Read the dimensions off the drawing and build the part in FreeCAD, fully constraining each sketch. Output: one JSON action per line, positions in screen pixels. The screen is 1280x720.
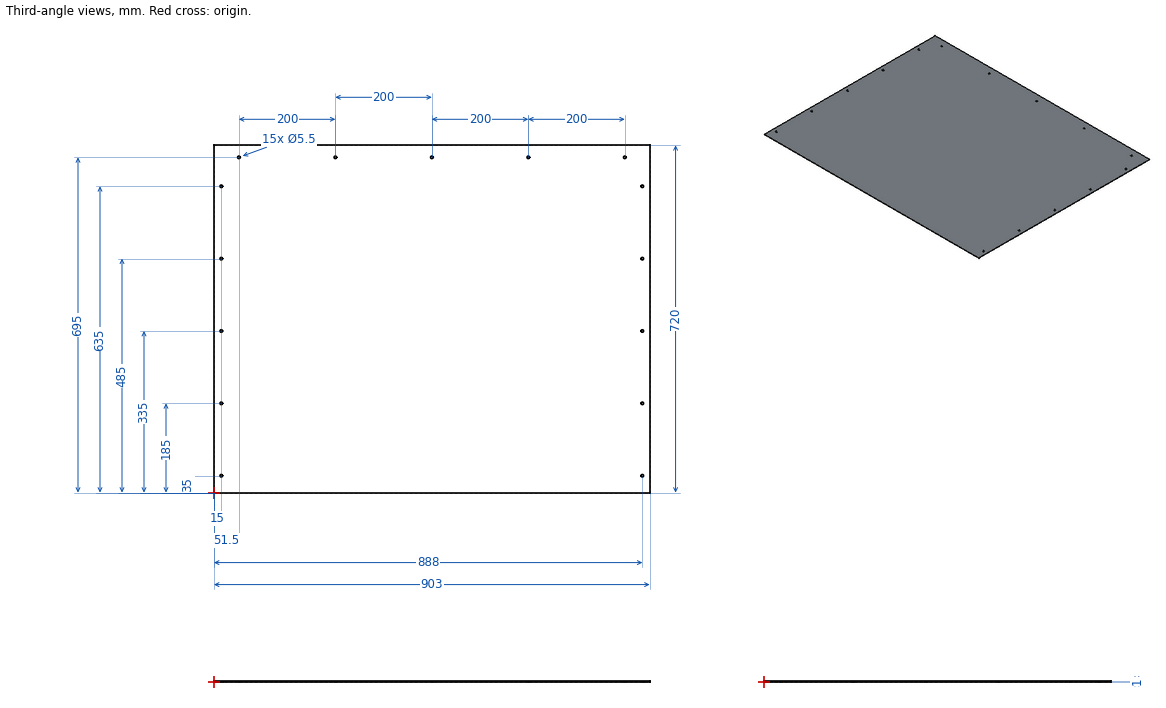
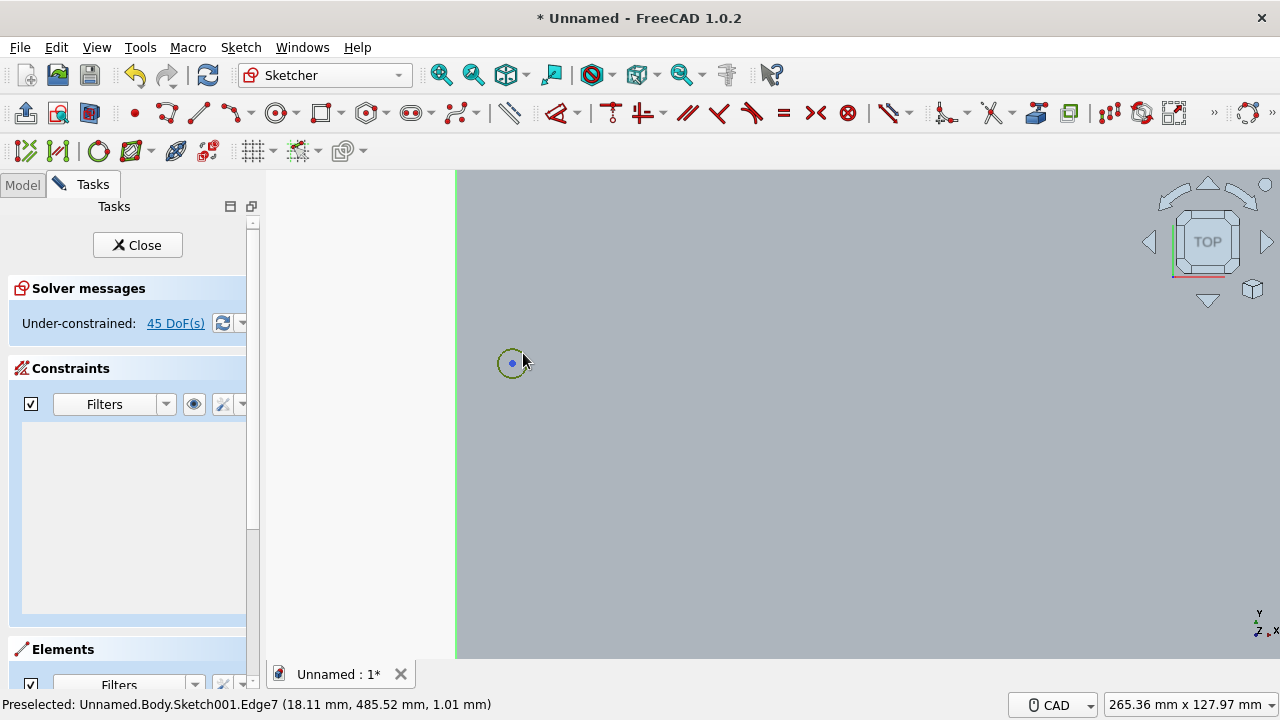
{"action": "scroll", "coordinate": [523, 357], "scroll_direction": "down", "scroll_amount": 11}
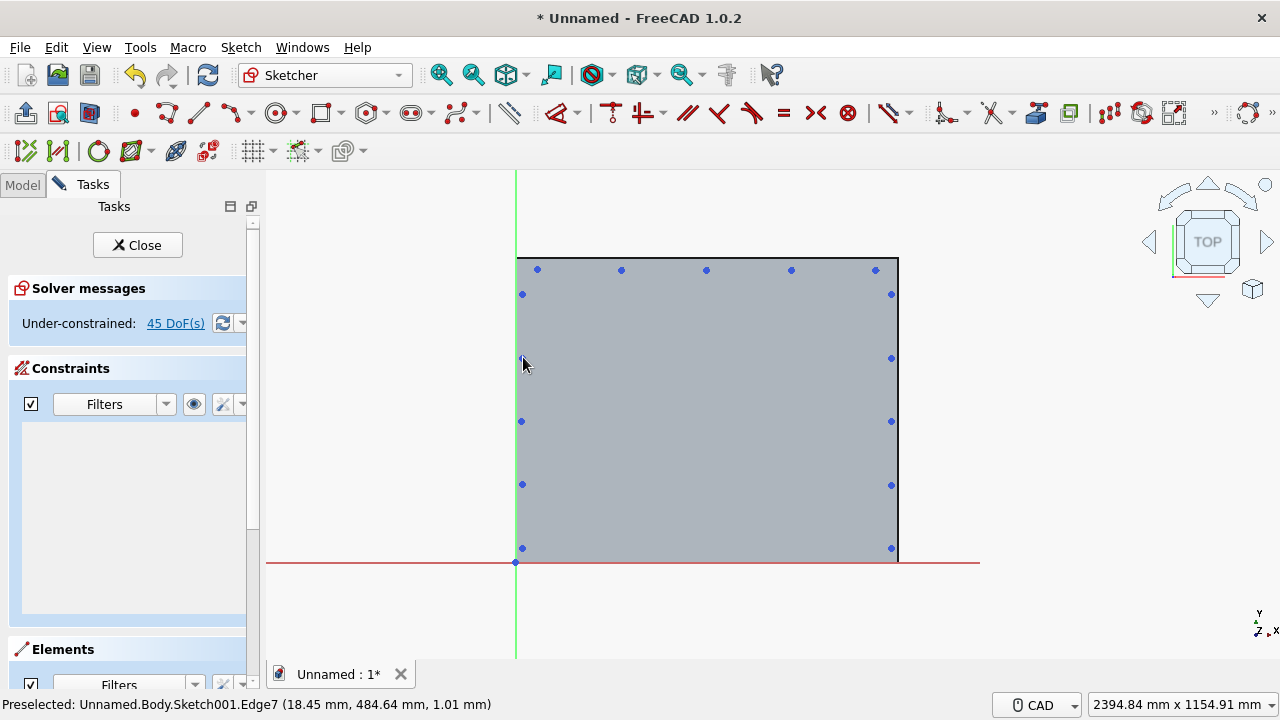
{"action": "scroll", "coordinate": [523, 420], "scroll_direction": "up", "scroll_amount": 12}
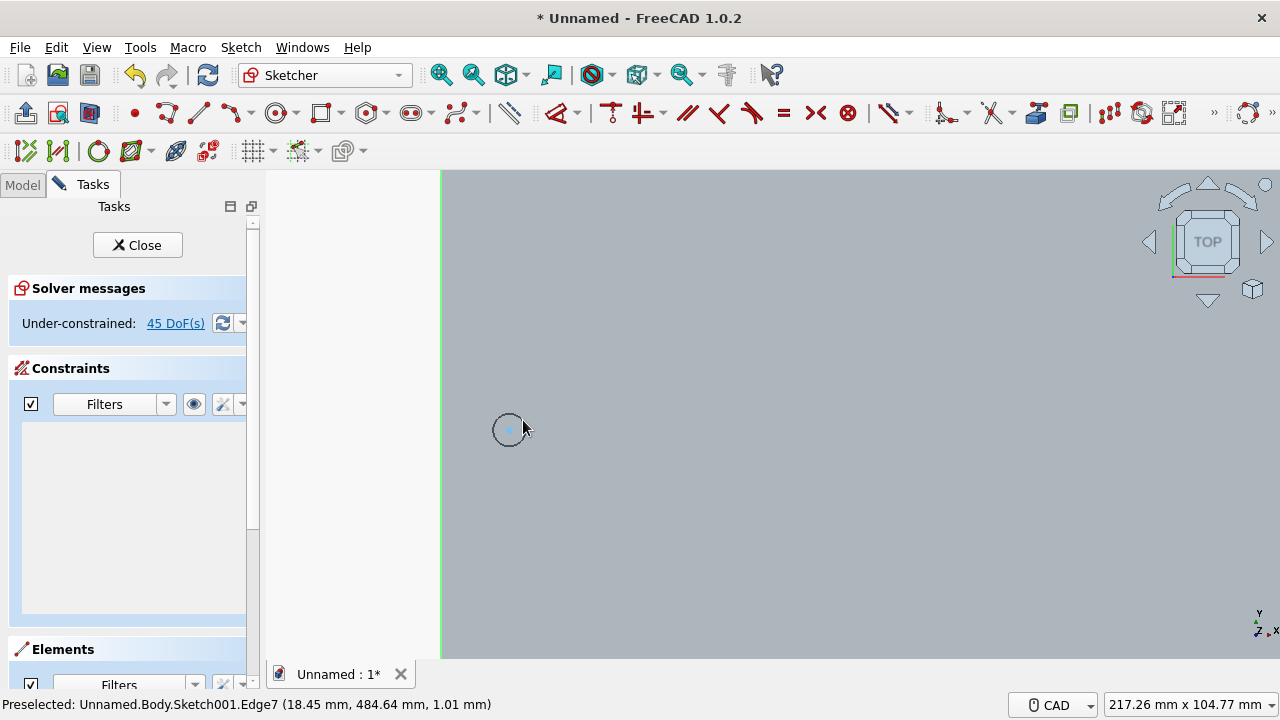
{"action": "left_click", "coordinate": [521, 419]}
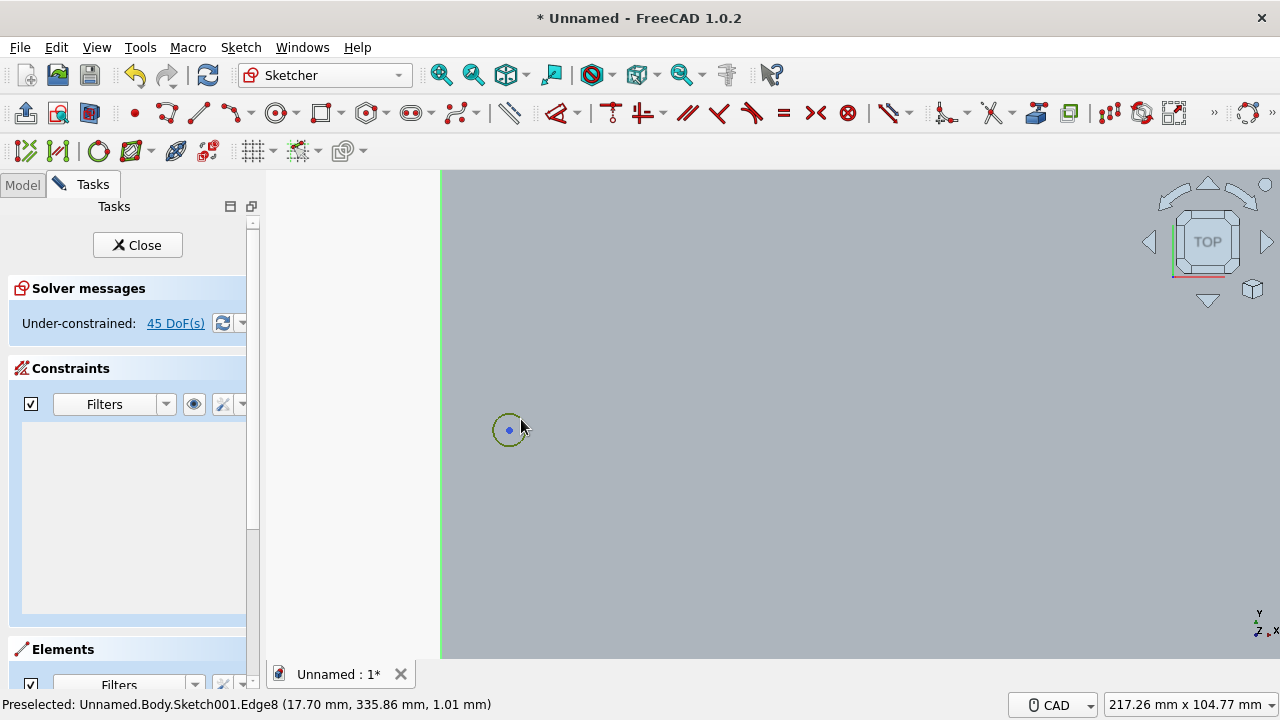
{"action": "scroll", "coordinate": [523, 420], "scroll_direction": "down", "scroll_amount": 12}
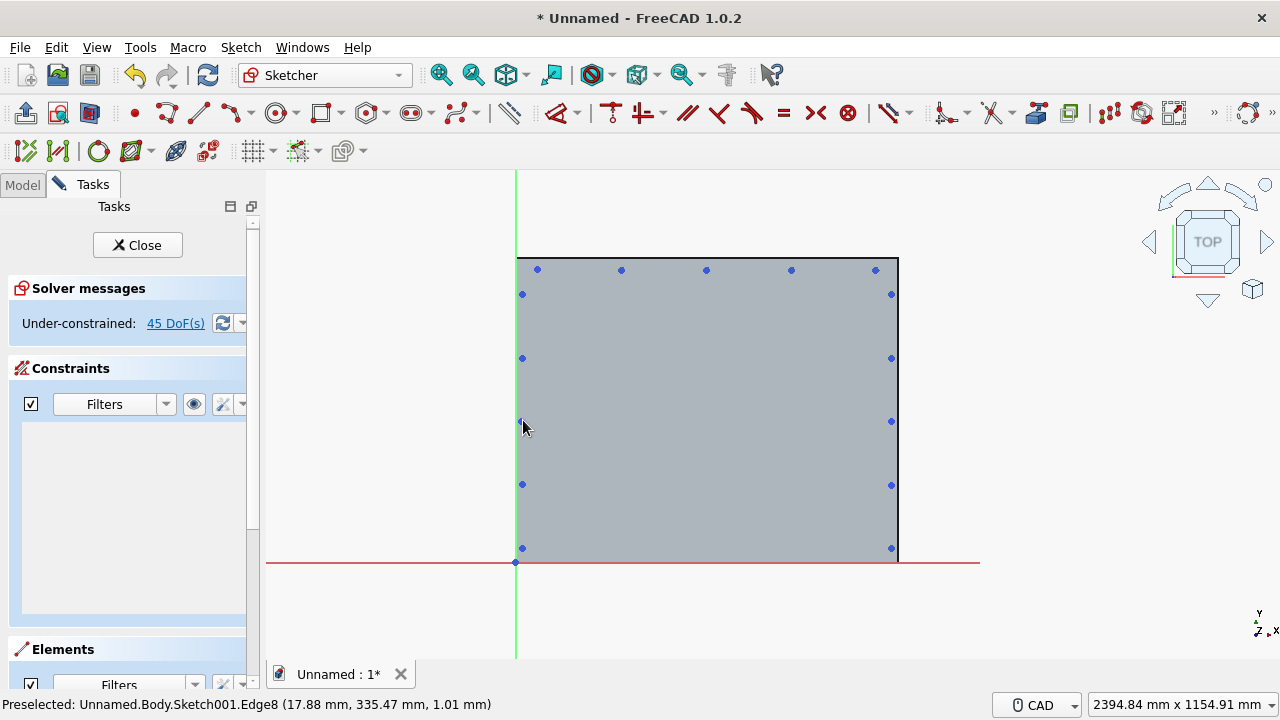
{"action": "scroll", "coordinate": [523, 484], "scroll_direction": "up", "scroll_amount": 12}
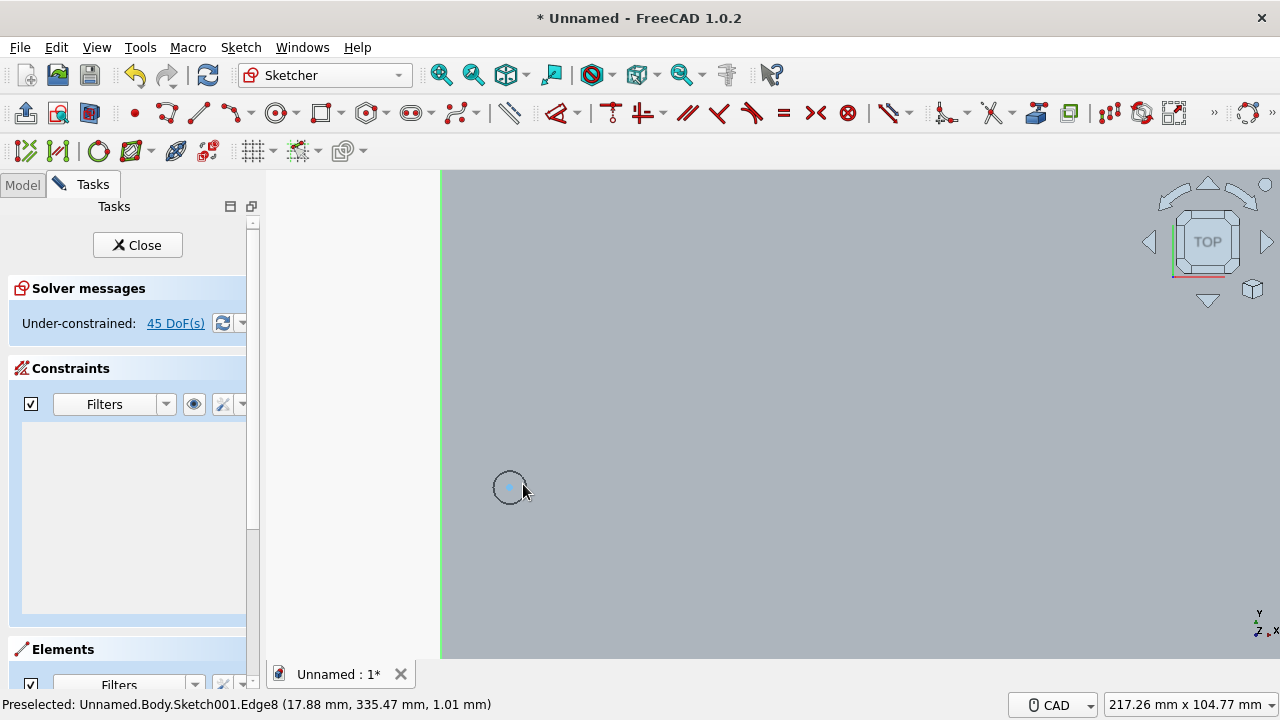
{"action": "left_click", "coordinate": [521, 476]}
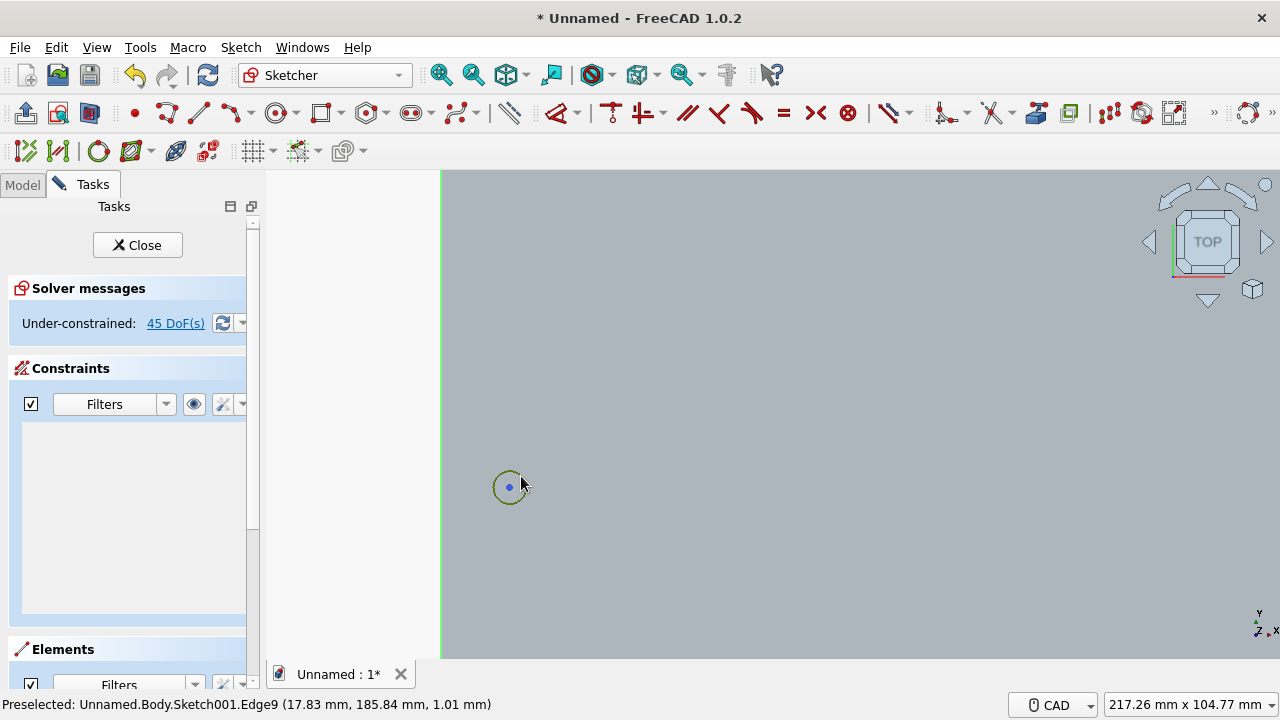
{"action": "scroll", "coordinate": [523, 484], "scroll_direction": "down", "scroll_amount": 12}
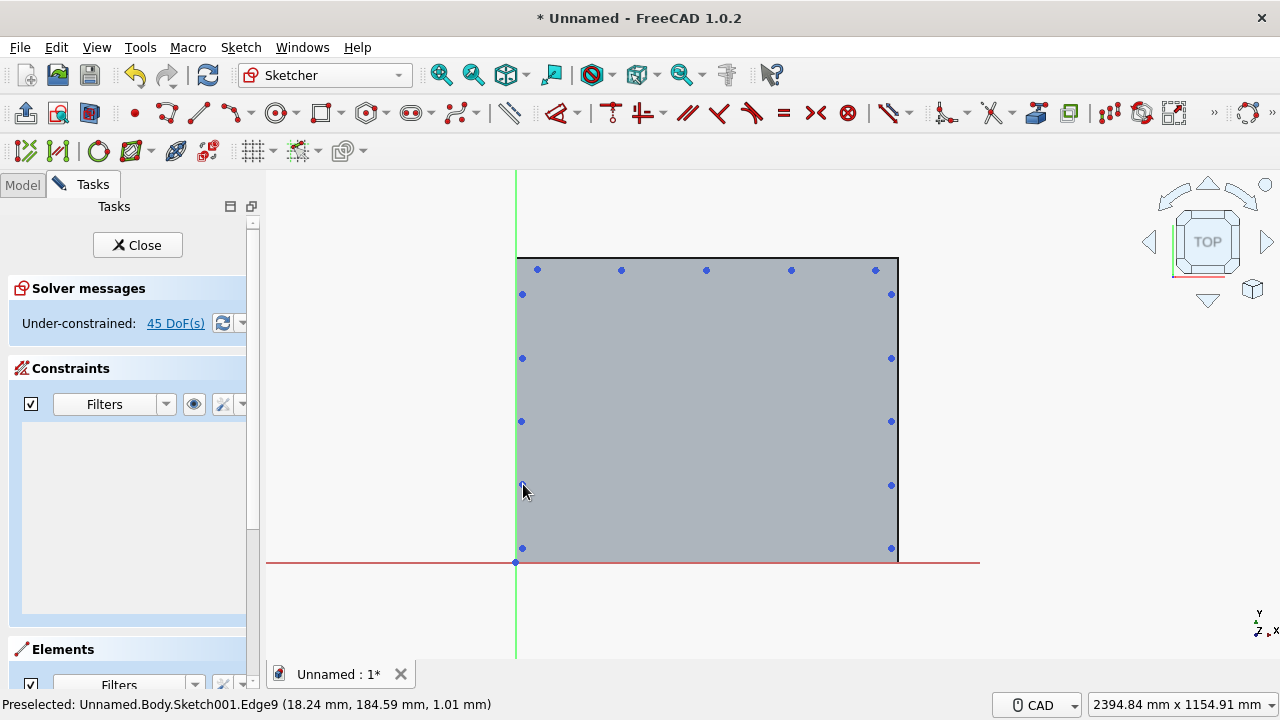
{"action": "scroll", "coordinate": [523, 547], "scroll_direction": "up", "scroll_amount": 12}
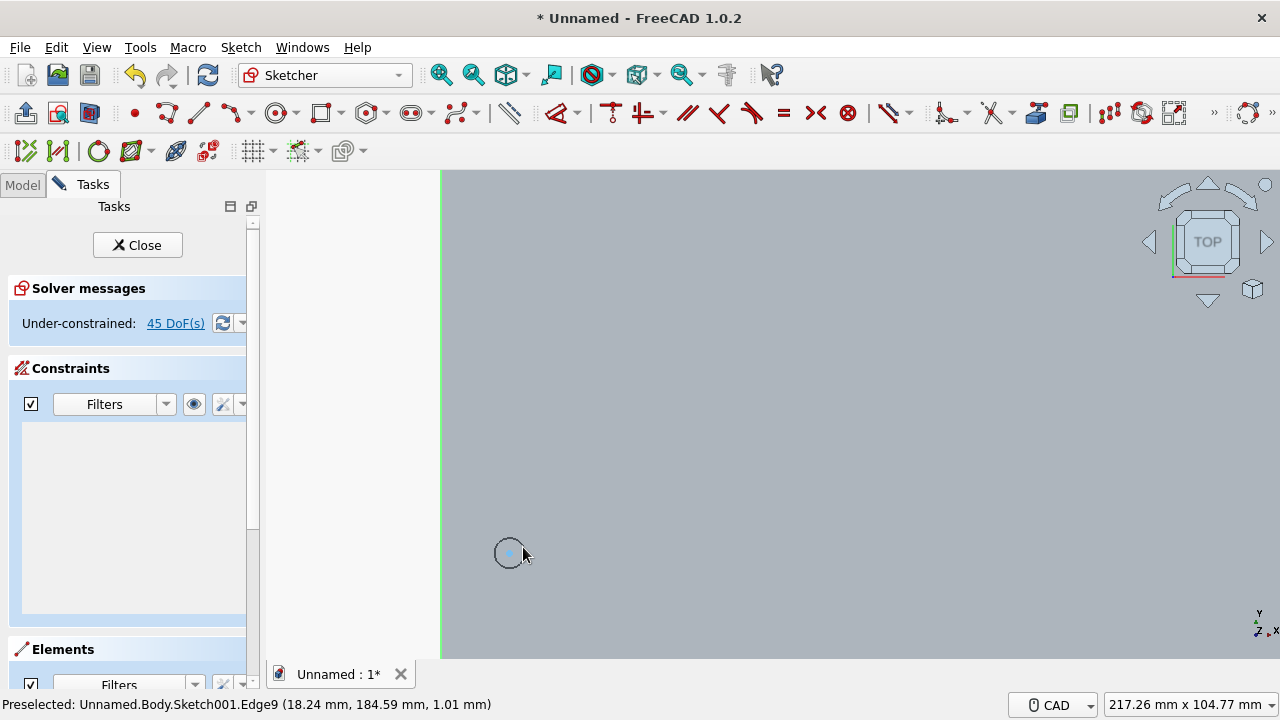
{"action": "left_click", "coordinate": [520, 543]}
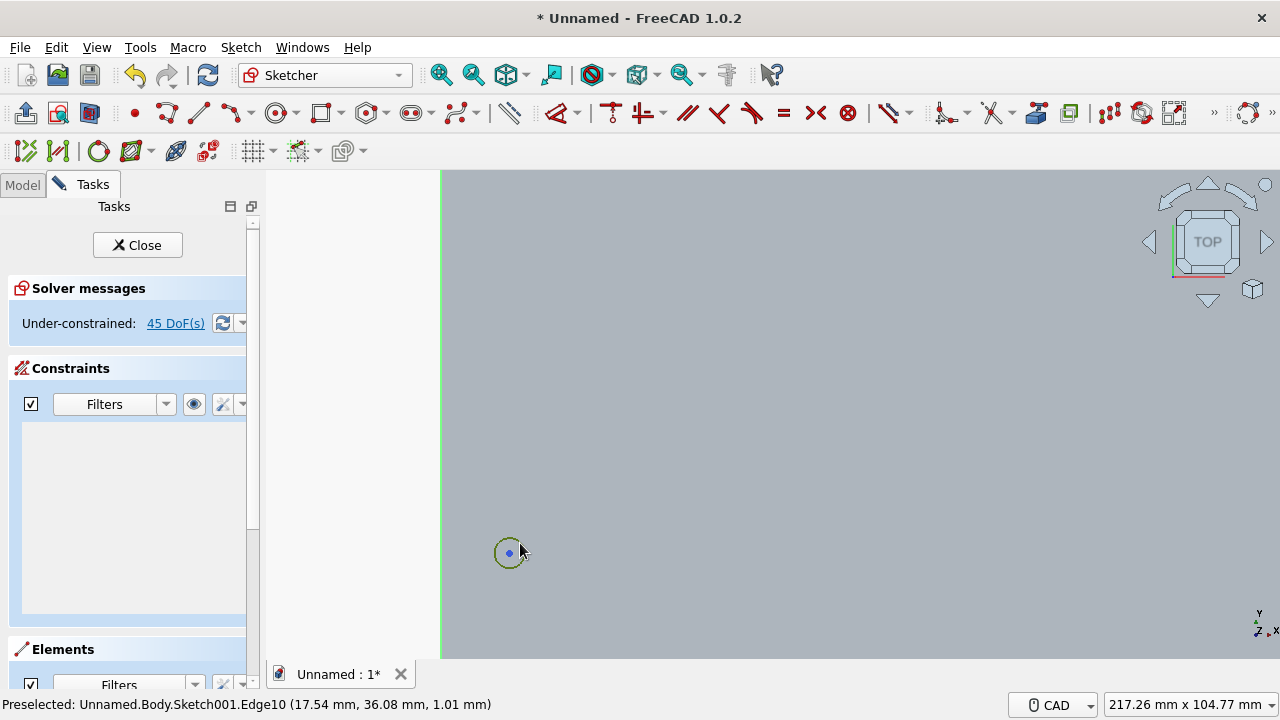
{"action": "scroll", "coordinate": [523, 547], "scroll_direction": "down", "scroll_amount": 12}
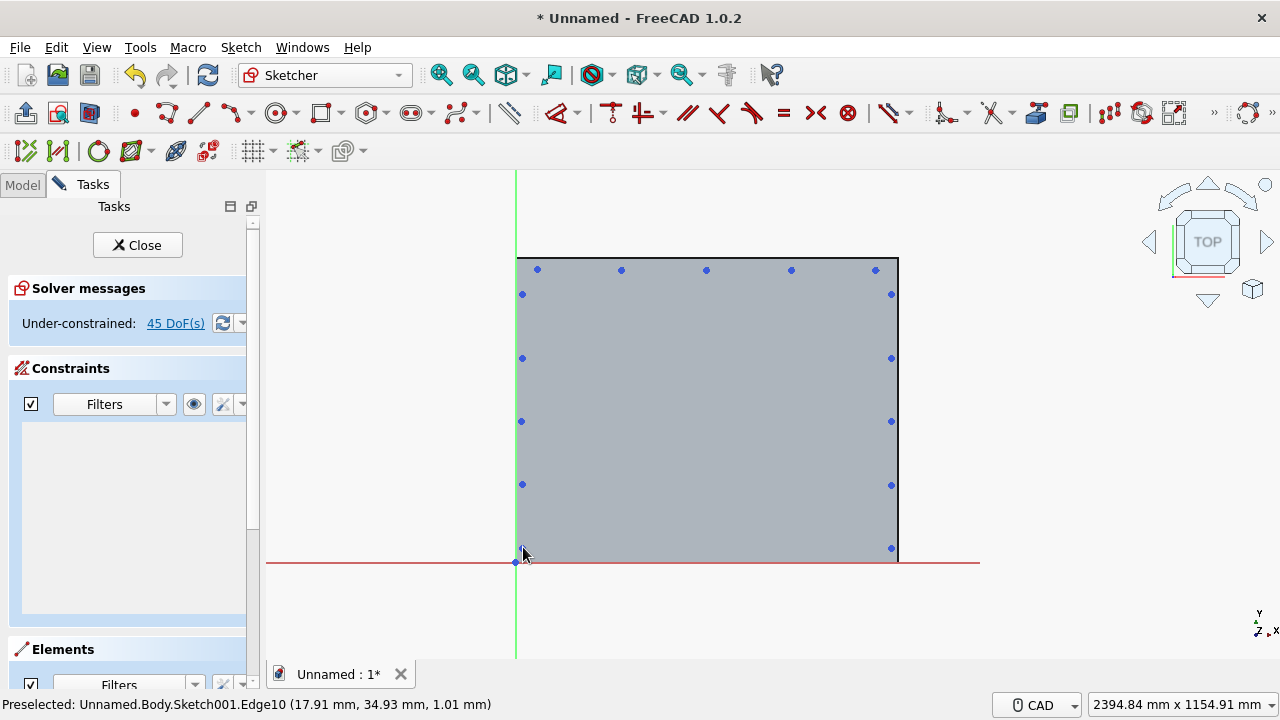
{"action": "scroll", "coordinate": [893, 548], "scroll_direction": "up", "scroll_amount": 11}